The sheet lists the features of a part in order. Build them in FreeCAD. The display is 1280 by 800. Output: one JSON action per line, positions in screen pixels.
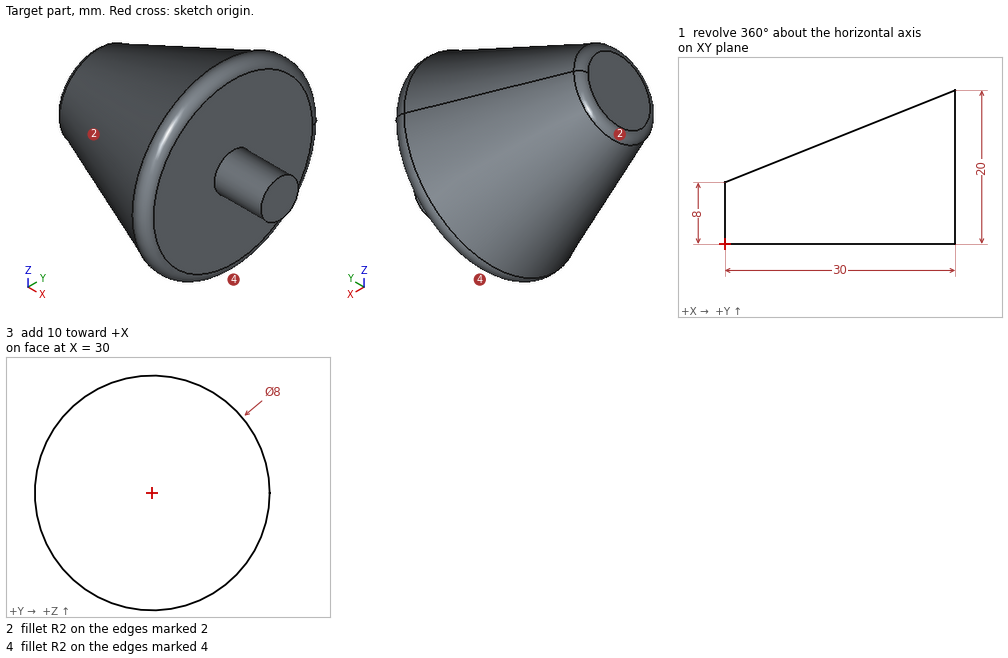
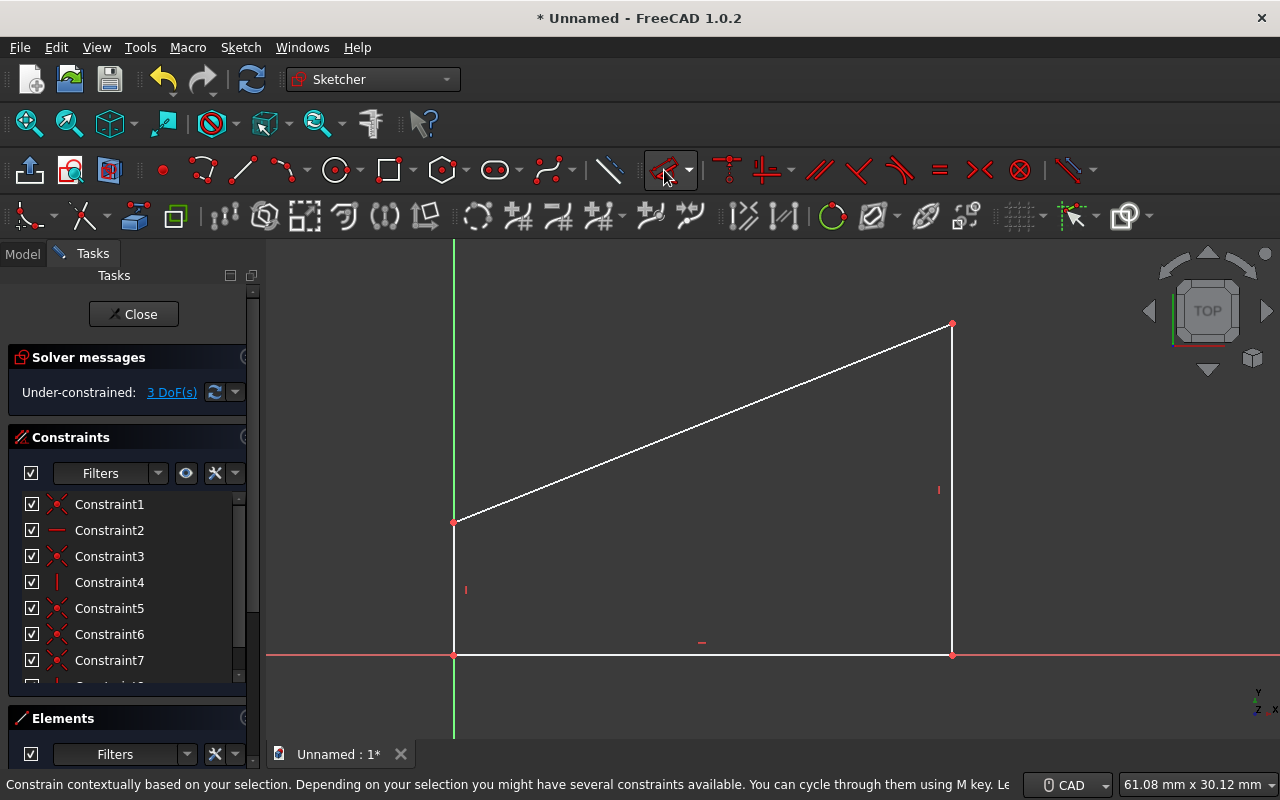
{"action": "left_click", "coordinate": [454, 563]}
{"action": "left_click", "coordinate": [420, 589]}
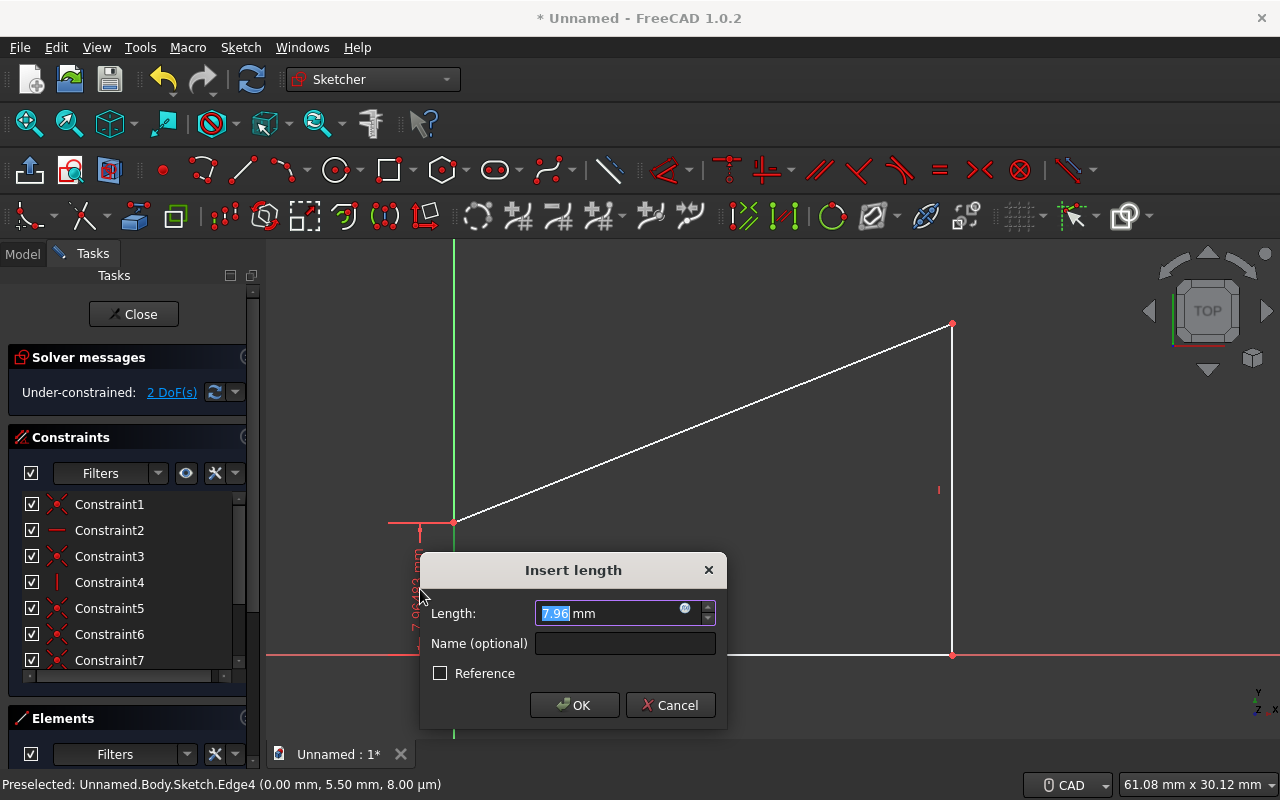
{"action": "type", "text": "8"}
{"action": "key", "text": "Return"}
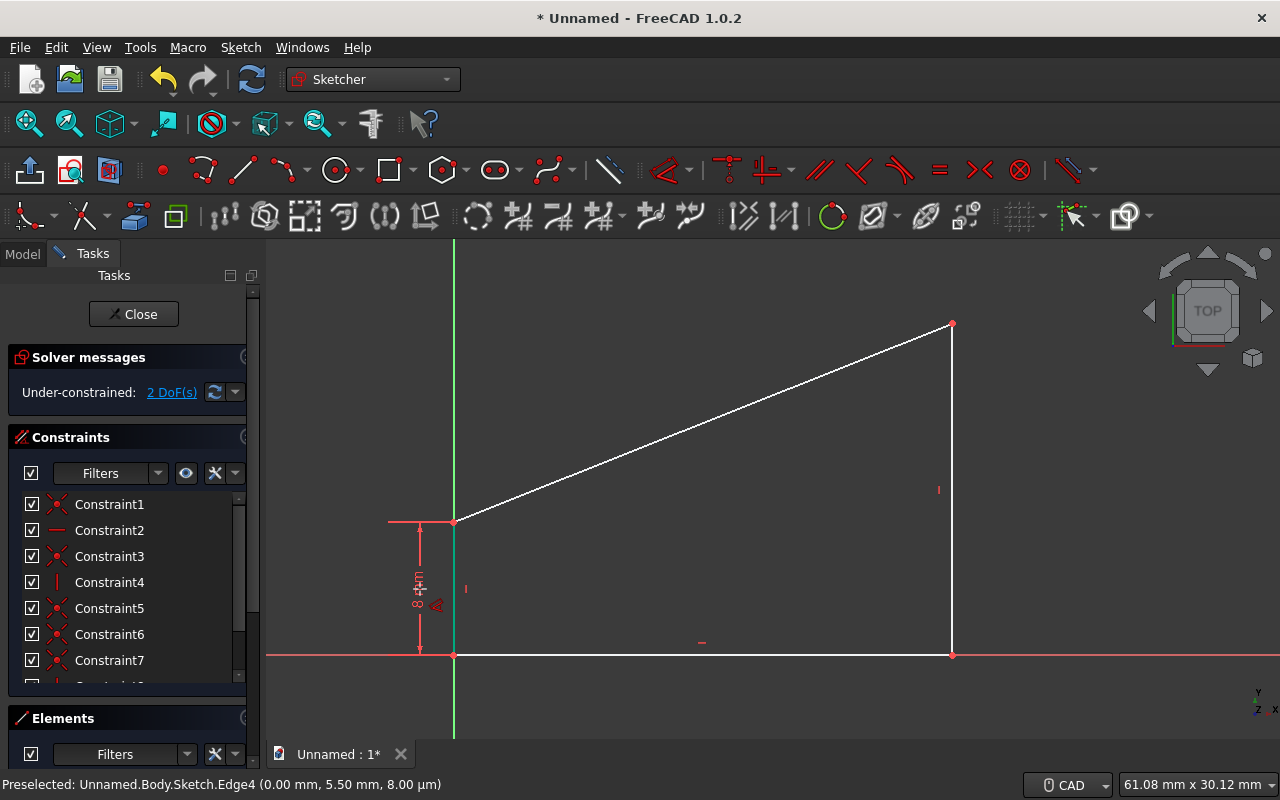
{"action": "left_click", "coordinate": [603, 655]}
{"action": "left_click", "coordinate": [703, 689]}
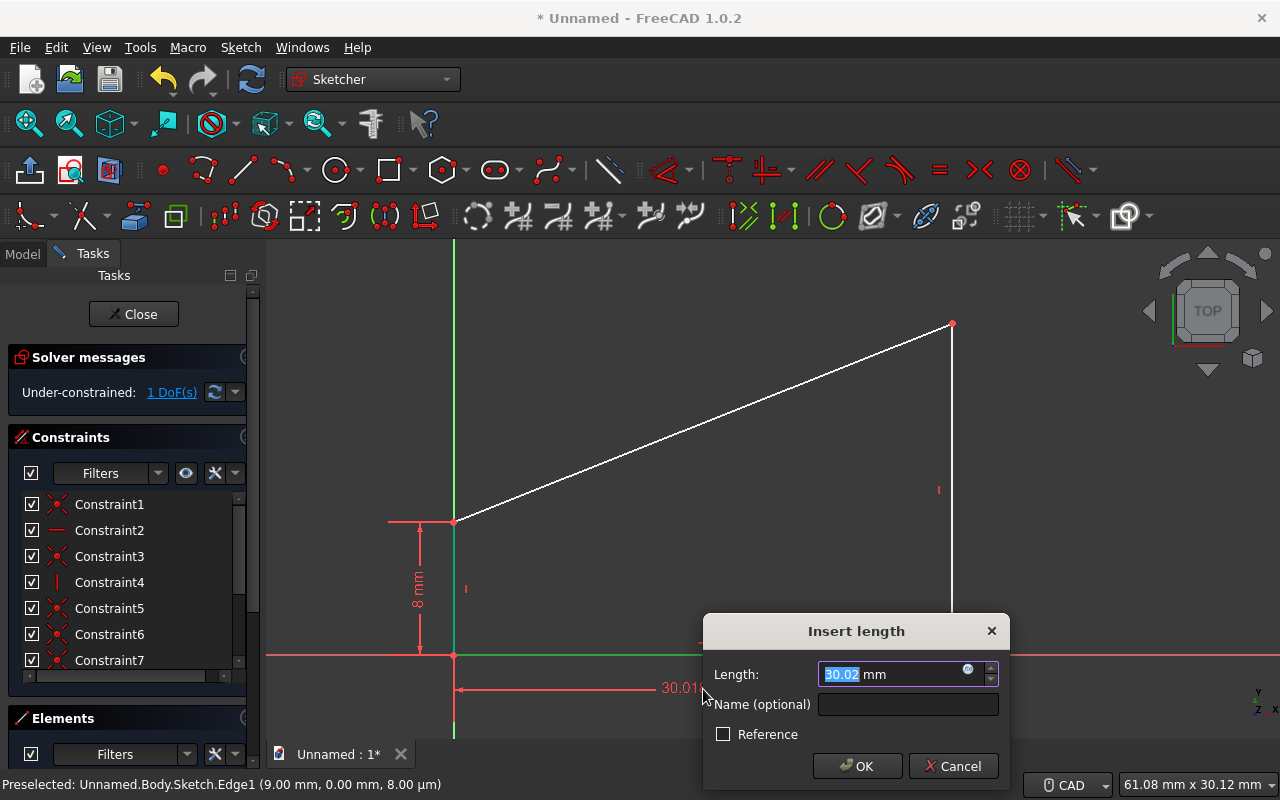
{"action": "type", "text": "30"}
{"action": "key", "text": "Return"}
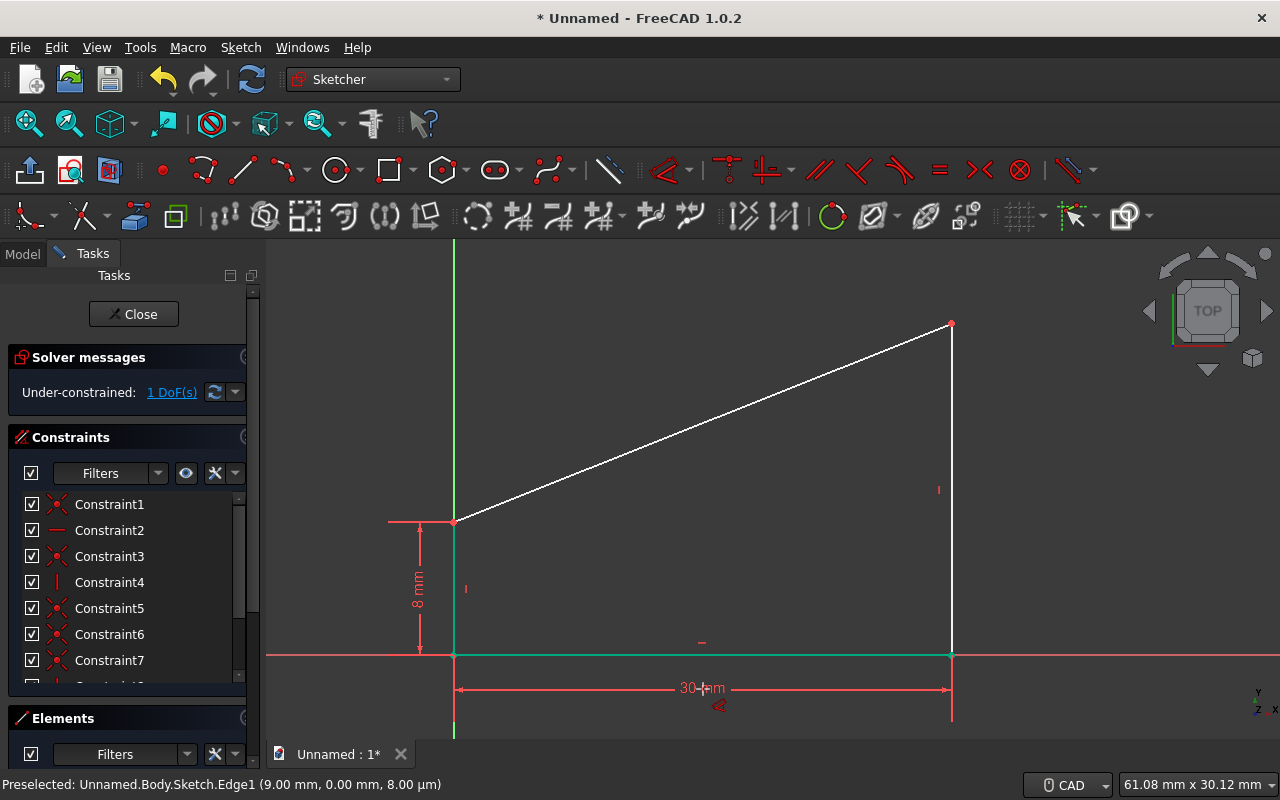
{"action": "left_click", "coordinate": [952, 556]}
{"action": "left_click", "coordinate": [986, 490]}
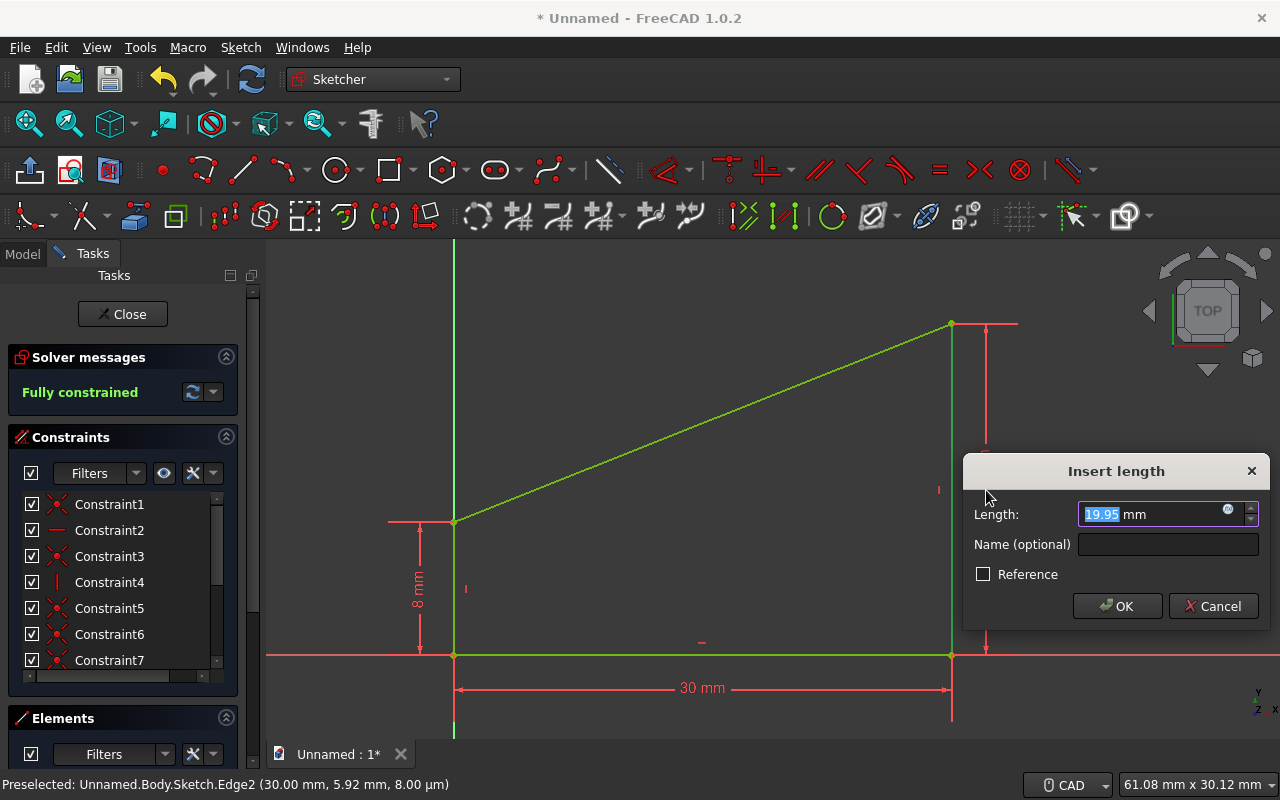
{"action": "type", "text": "20"}
{"action": "key", "text": "Return"}
{"action": "key", "text": "Escape"}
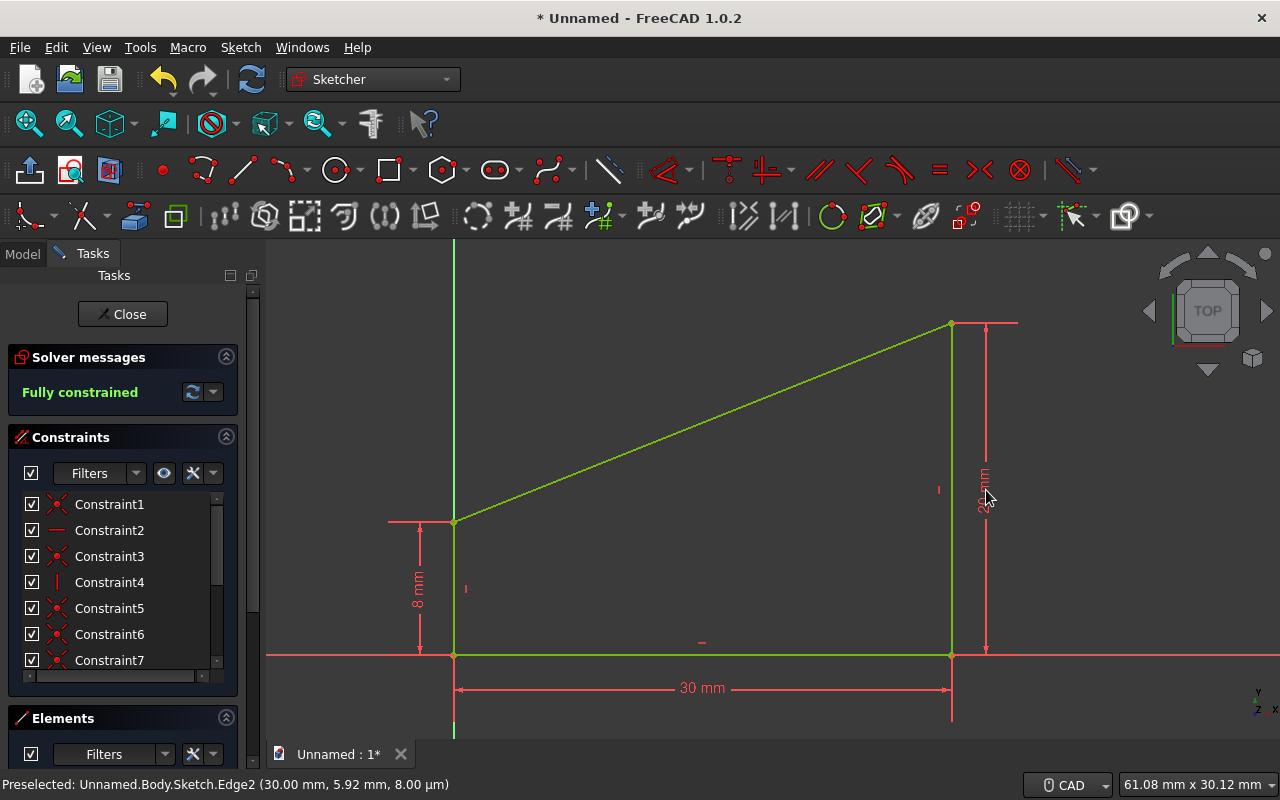
{"action": "left_click", "coordinate": [123, 314]}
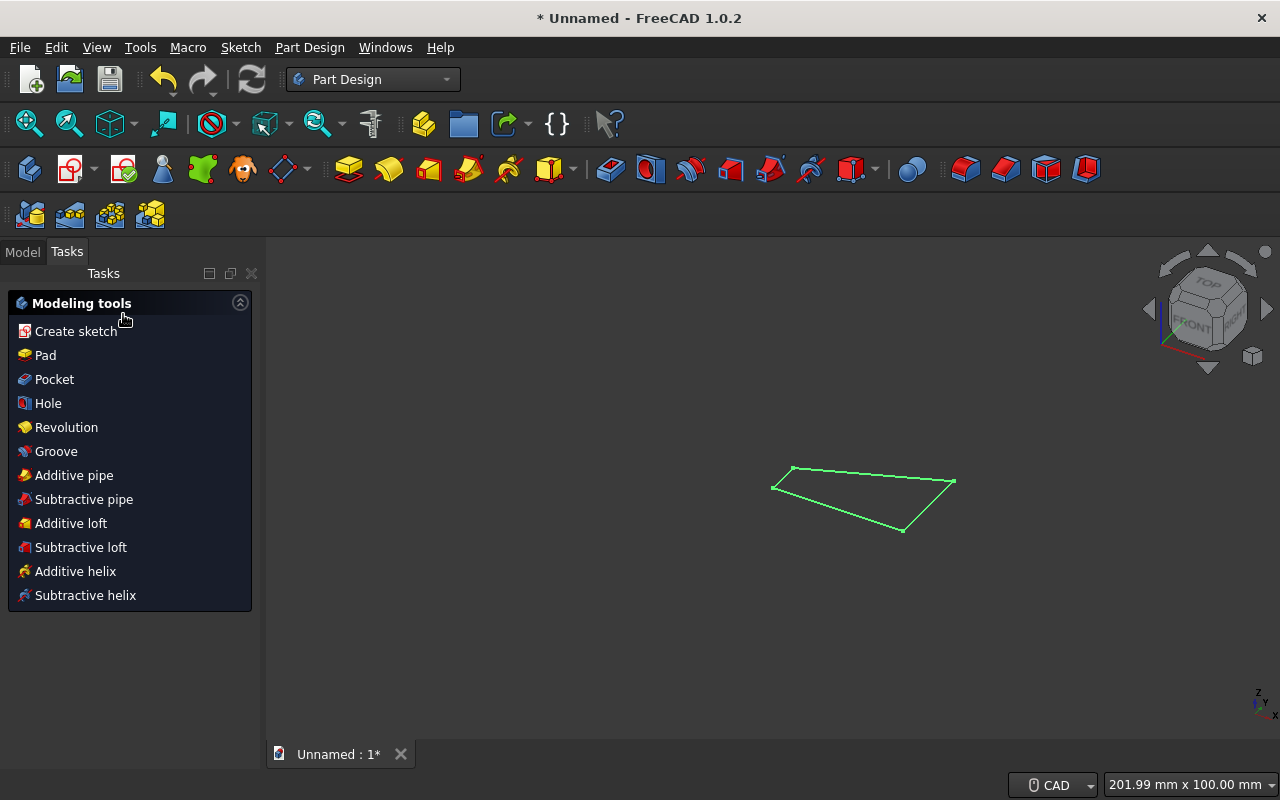
{"action": "left_click", "coordinate": [390, 170]}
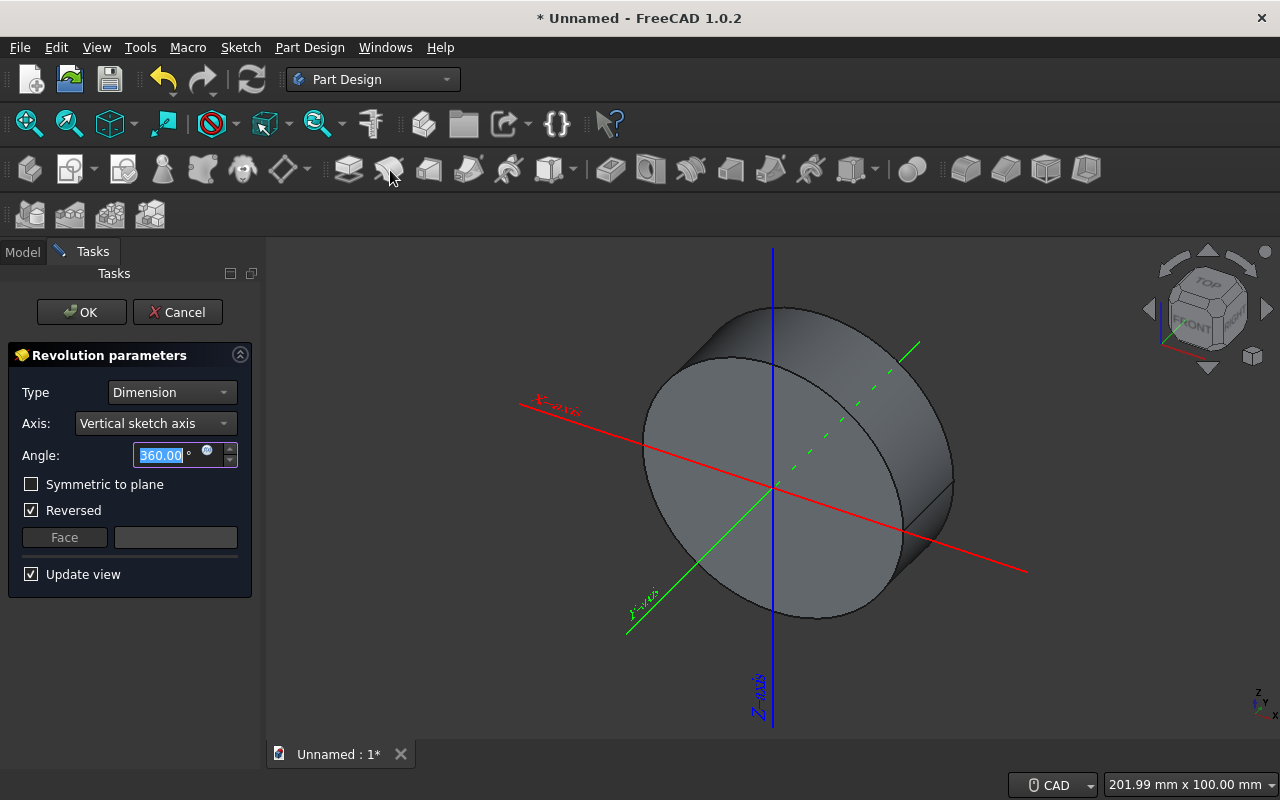
{"action": "left_click", "coordinate": [156, 424]}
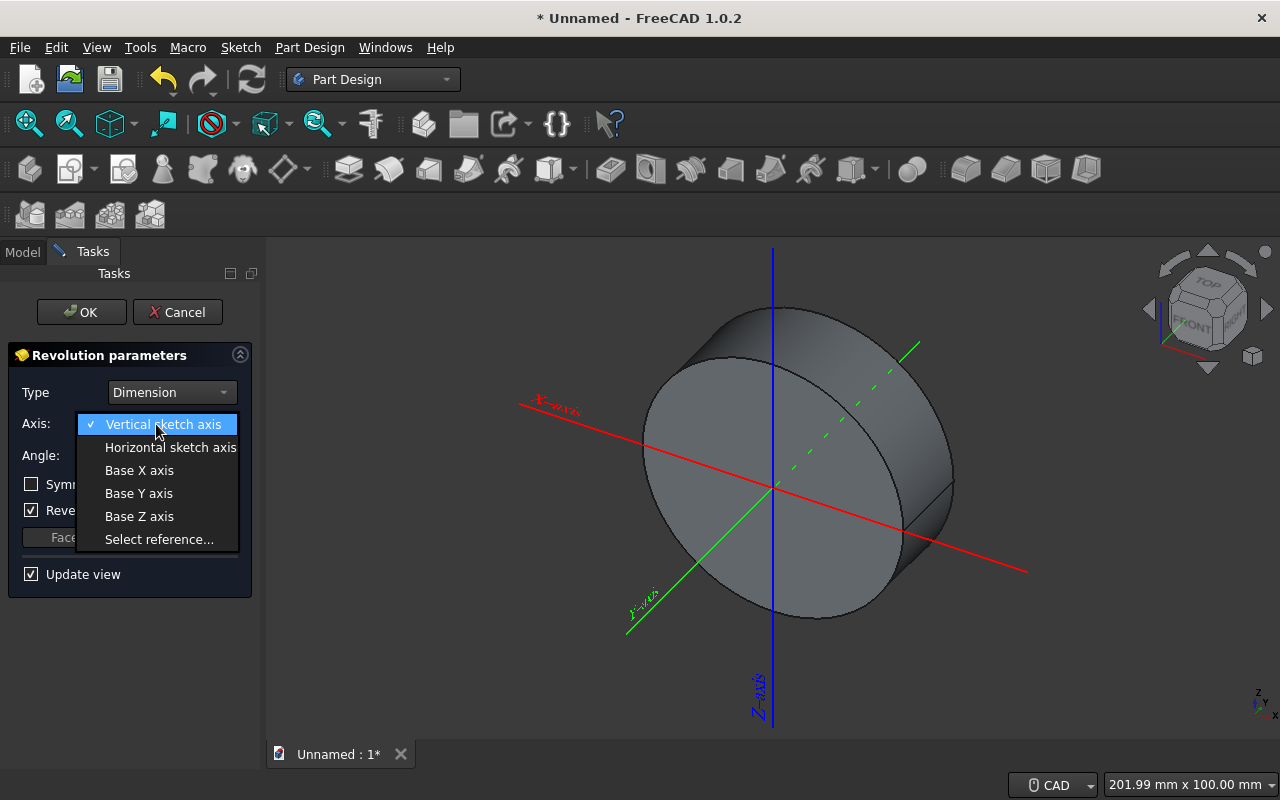
{"action": "left_click", "coordinate": [156, 448]}